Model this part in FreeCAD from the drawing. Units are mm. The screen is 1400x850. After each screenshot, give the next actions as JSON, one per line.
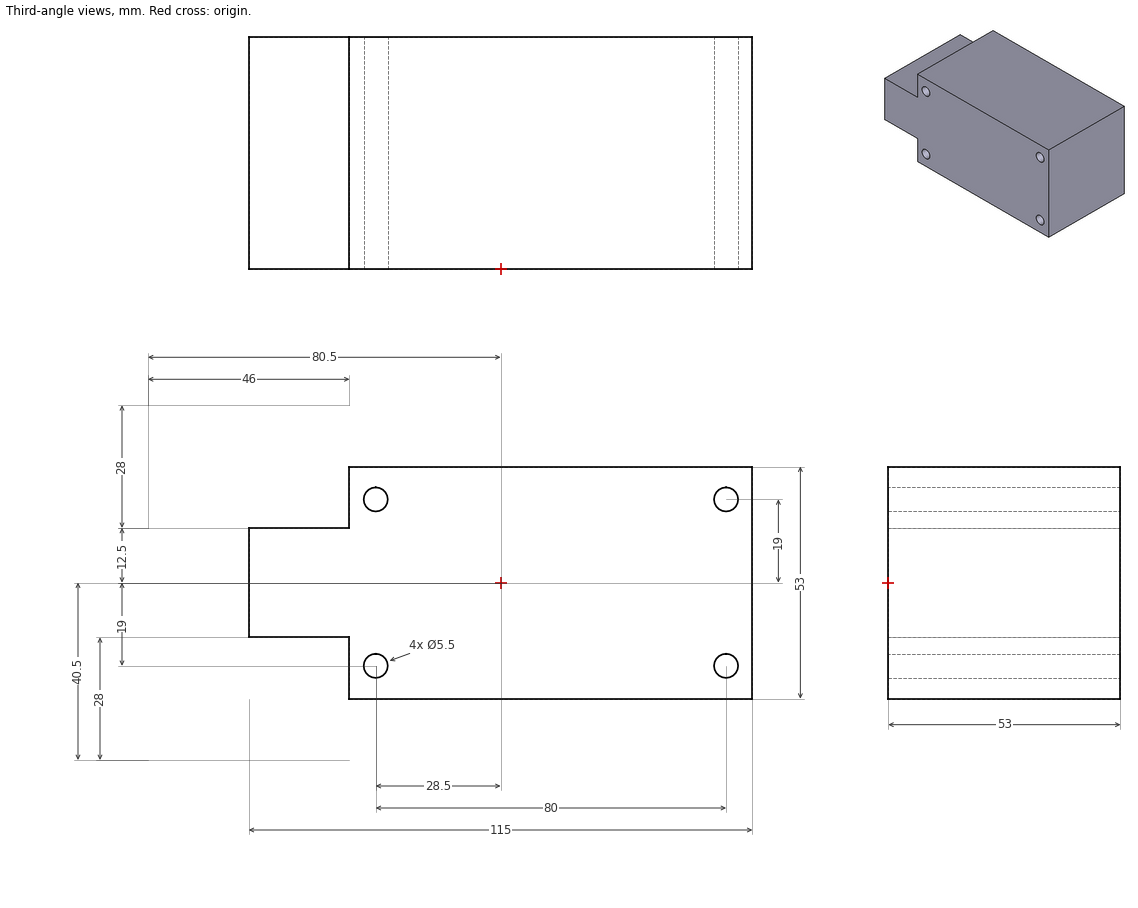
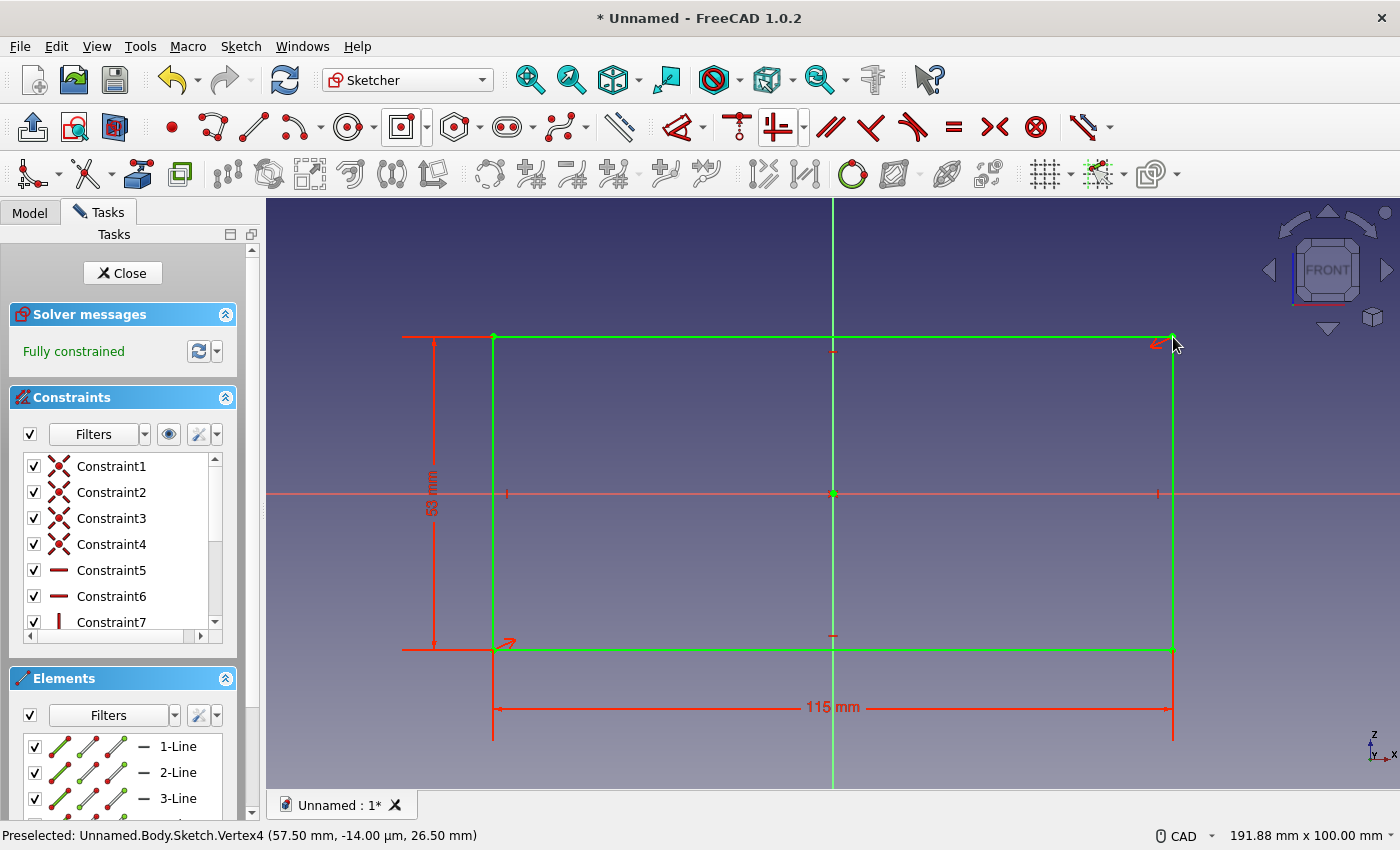
{"action": "left_click", "coordinate": [123, 273]}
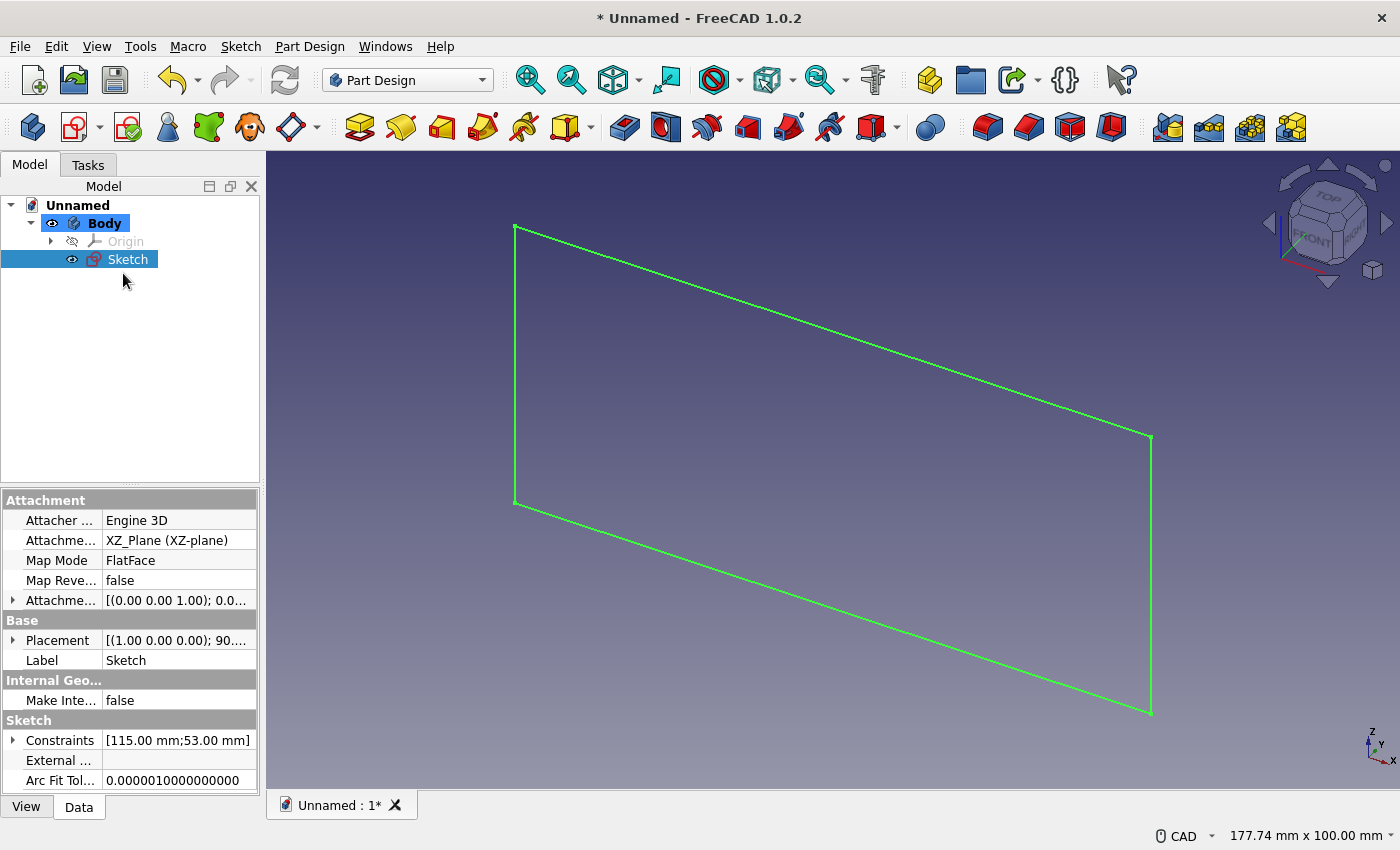
{"action": "left_click", "coordinate": [360, 128]}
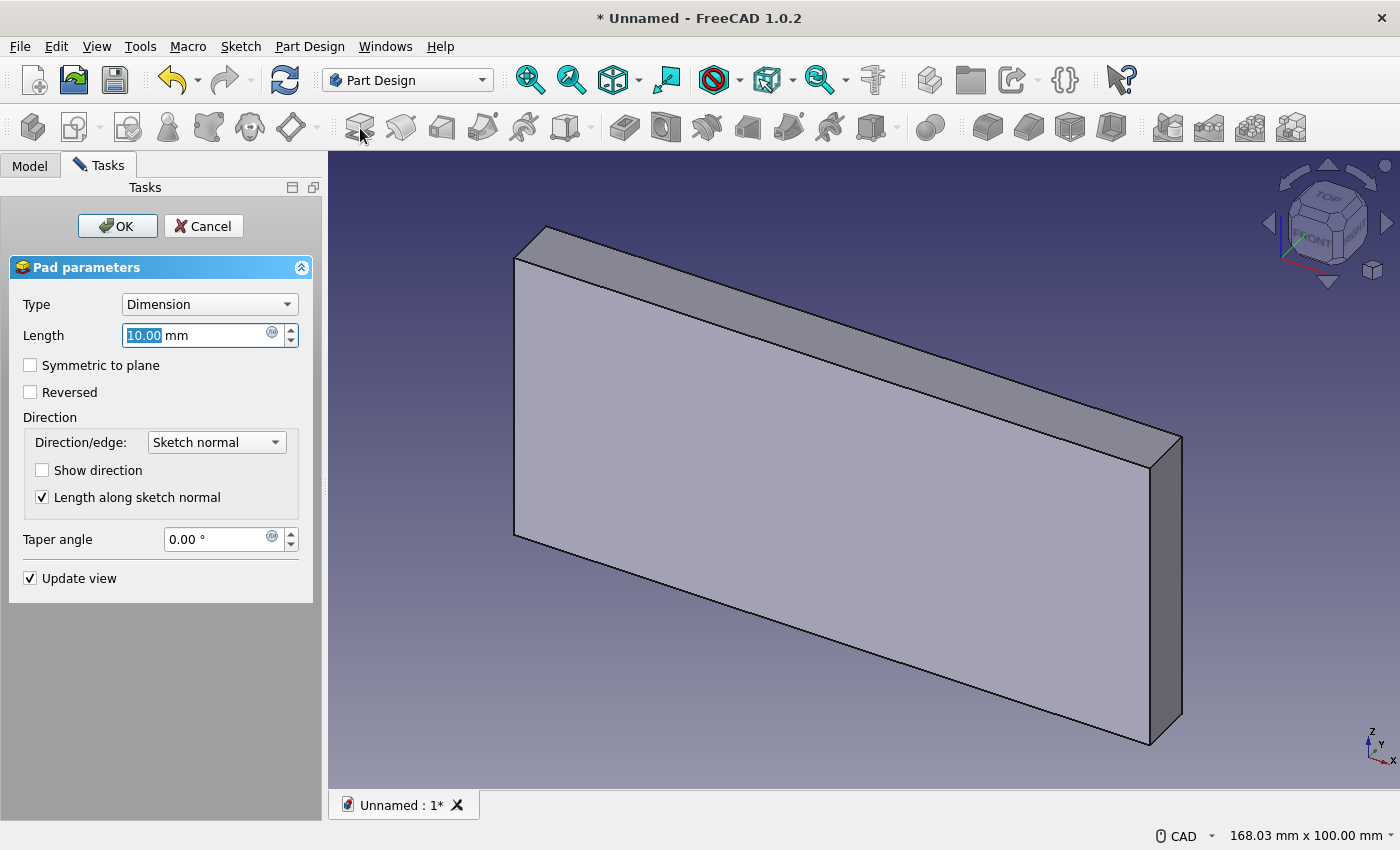
{"action": "type", "text": "53"}
{"action": "key", "text": "Tab"}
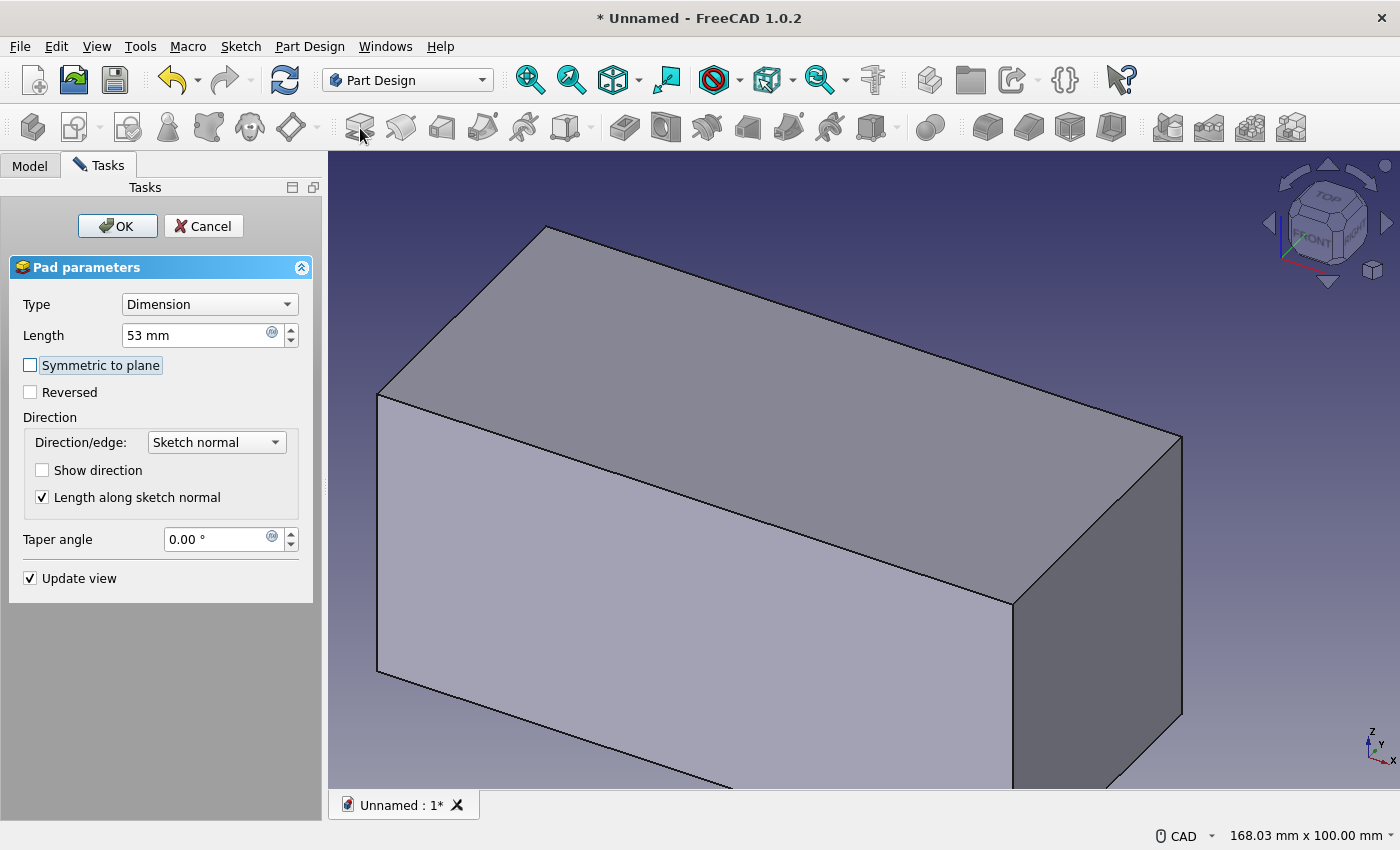
{"action": "left_click", "coordinate": [31, 392]}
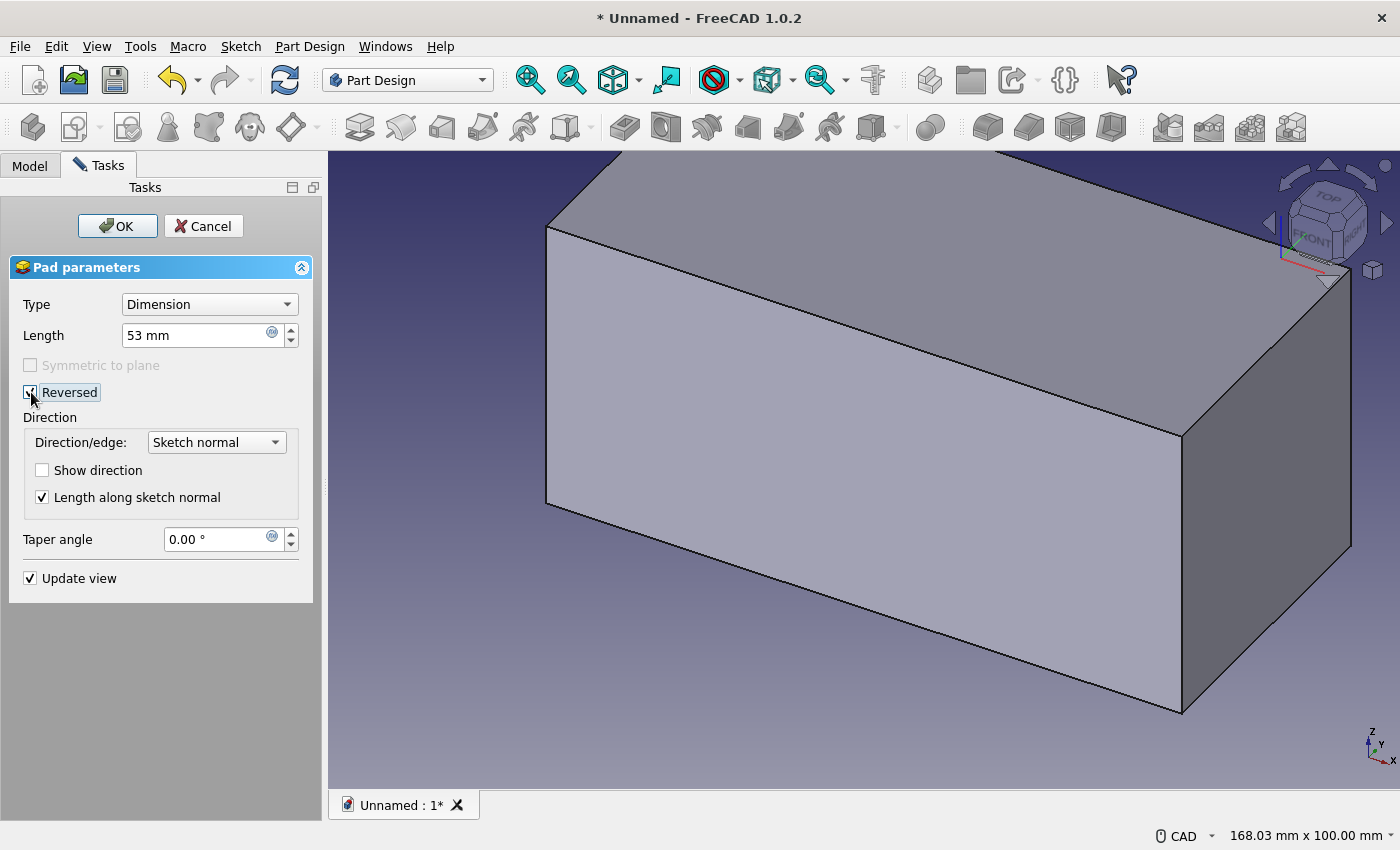
{"action": "left_click", "coordinate": [118, 226]}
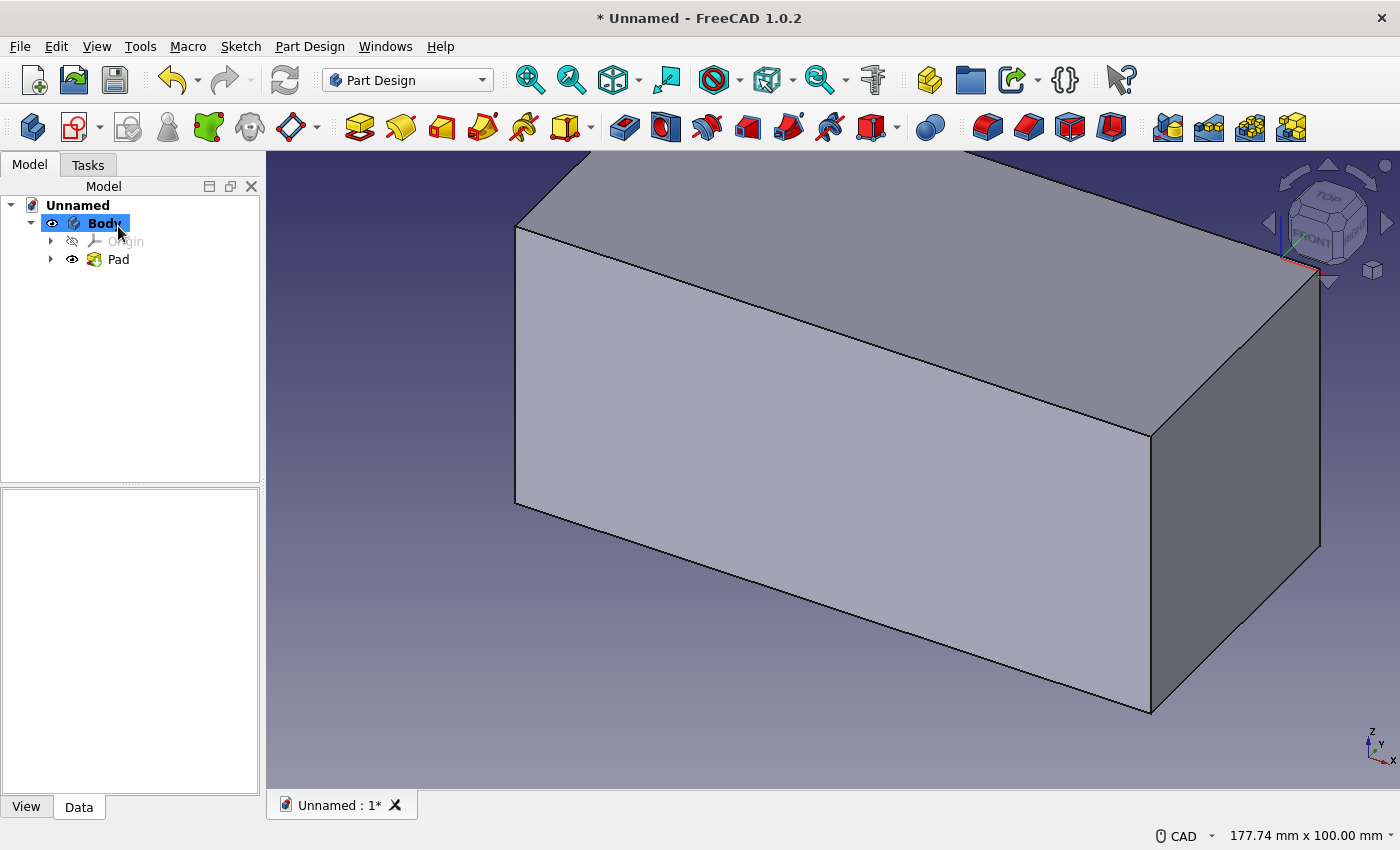
{"action": "left_click", "coordinate": [531, 80]}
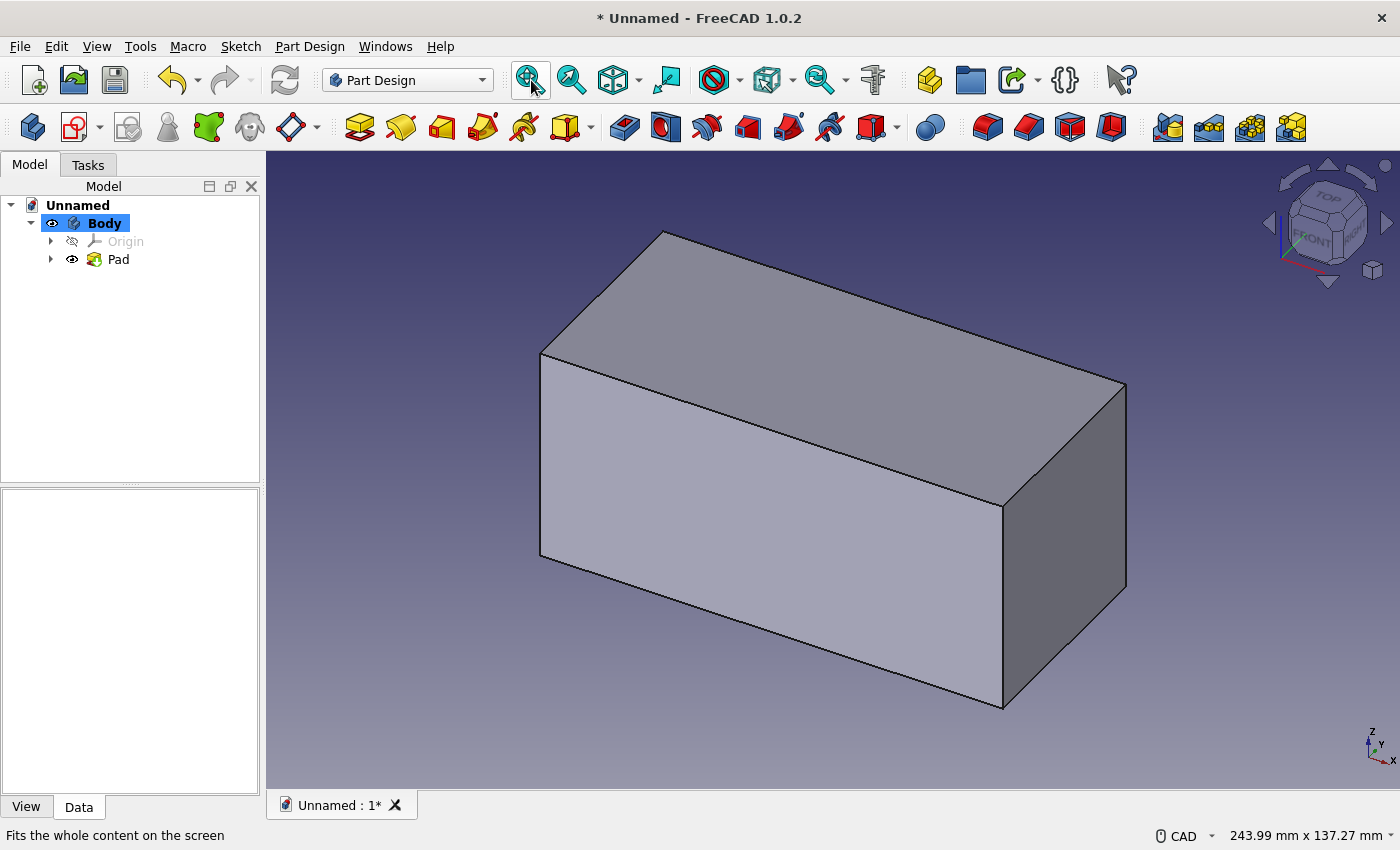
{"action": "key", "text": "4"}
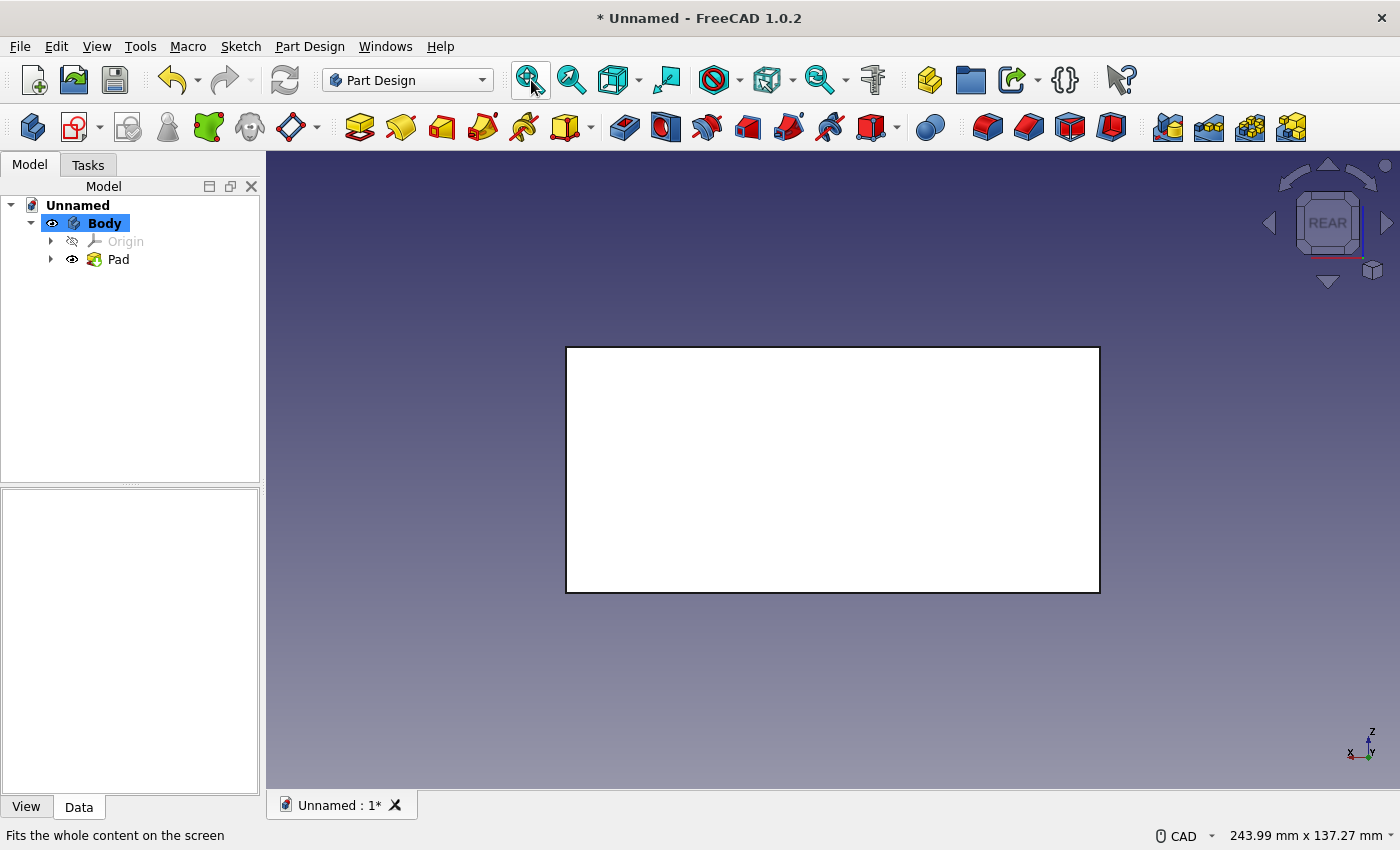
{"action": "left_click", "coordinate": [757, 469]}